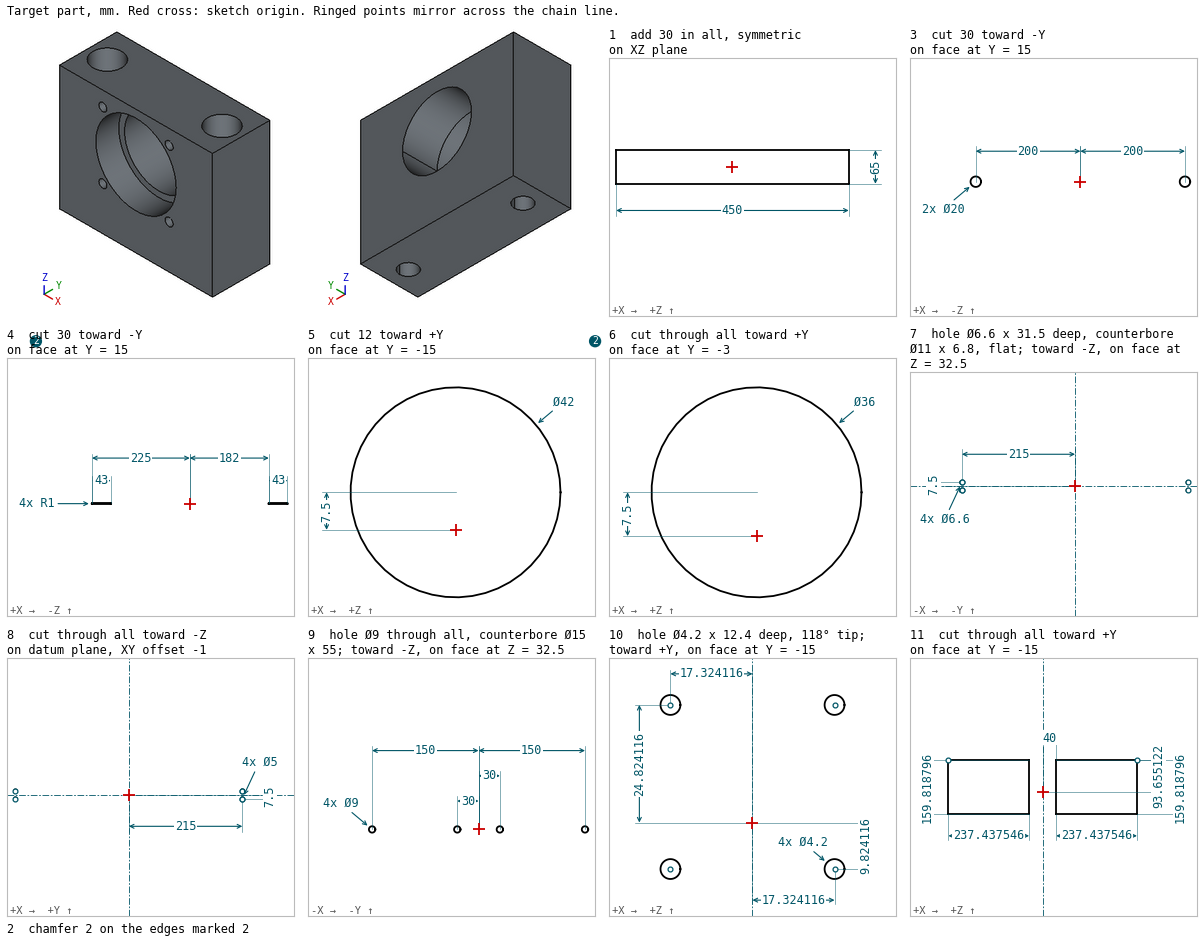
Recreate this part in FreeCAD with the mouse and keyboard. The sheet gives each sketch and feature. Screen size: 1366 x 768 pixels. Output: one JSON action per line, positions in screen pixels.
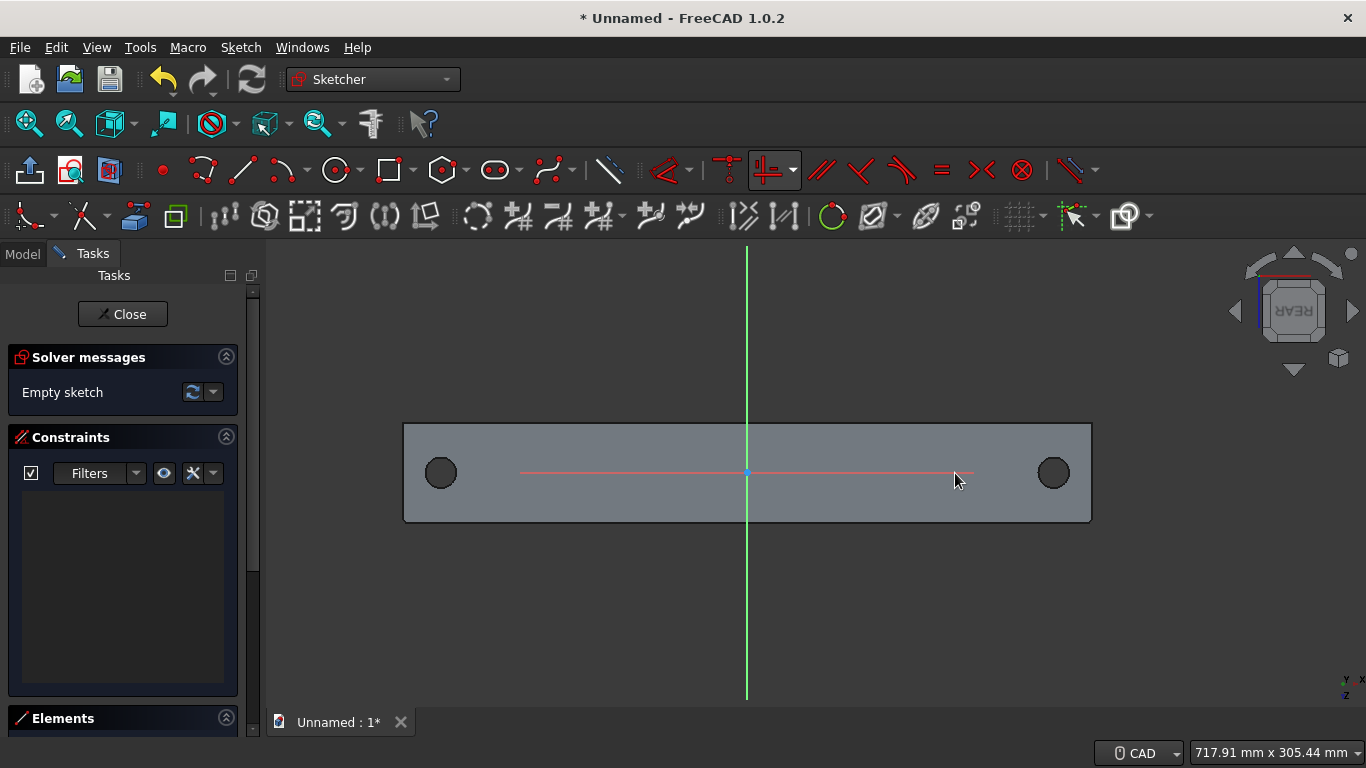
{"action": "scroll", "coordinate": [403, 473], "scroll_direction": "up", "scroll_amount": 14}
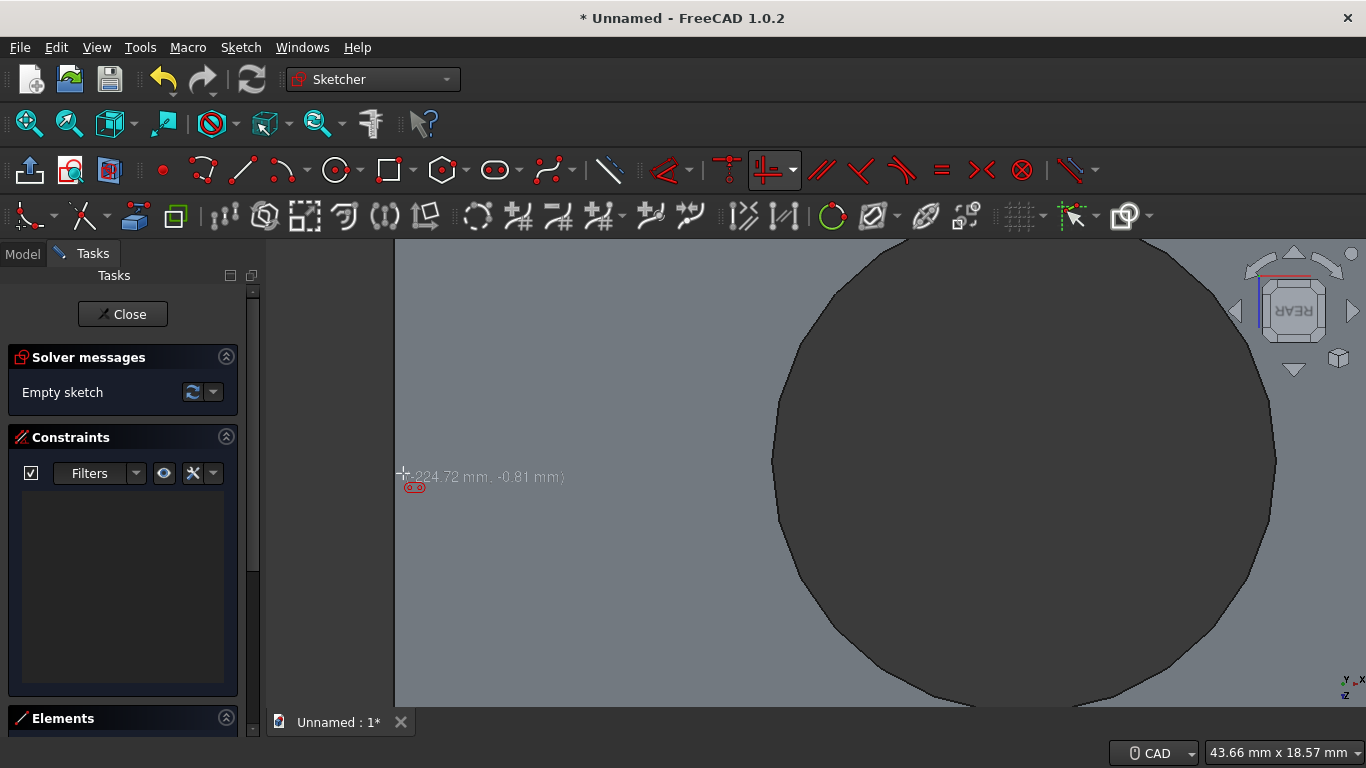
{"action": "scroll", "coordinate": [403, 474], "scroll_direction": "down", "scroll_amount": 14}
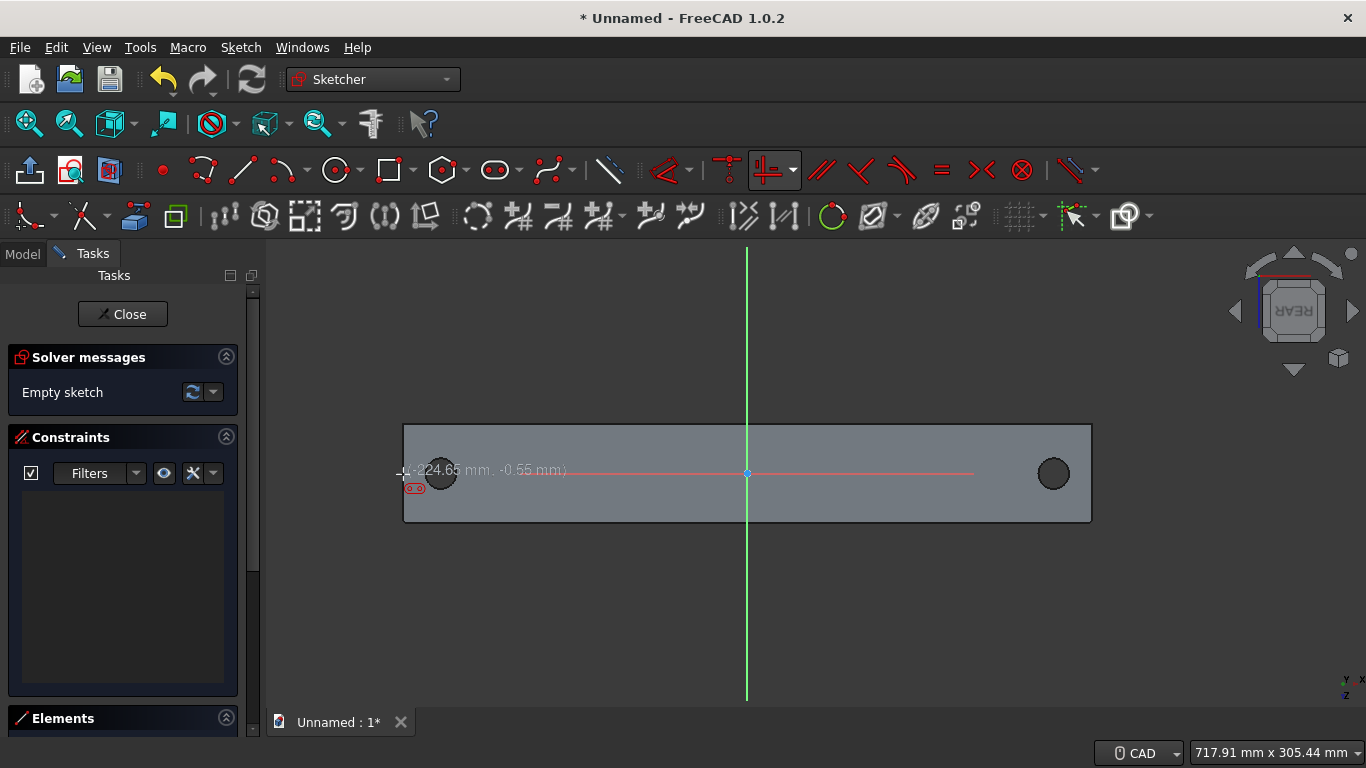
{"action": "left_click", "coordinate": [403, 474]}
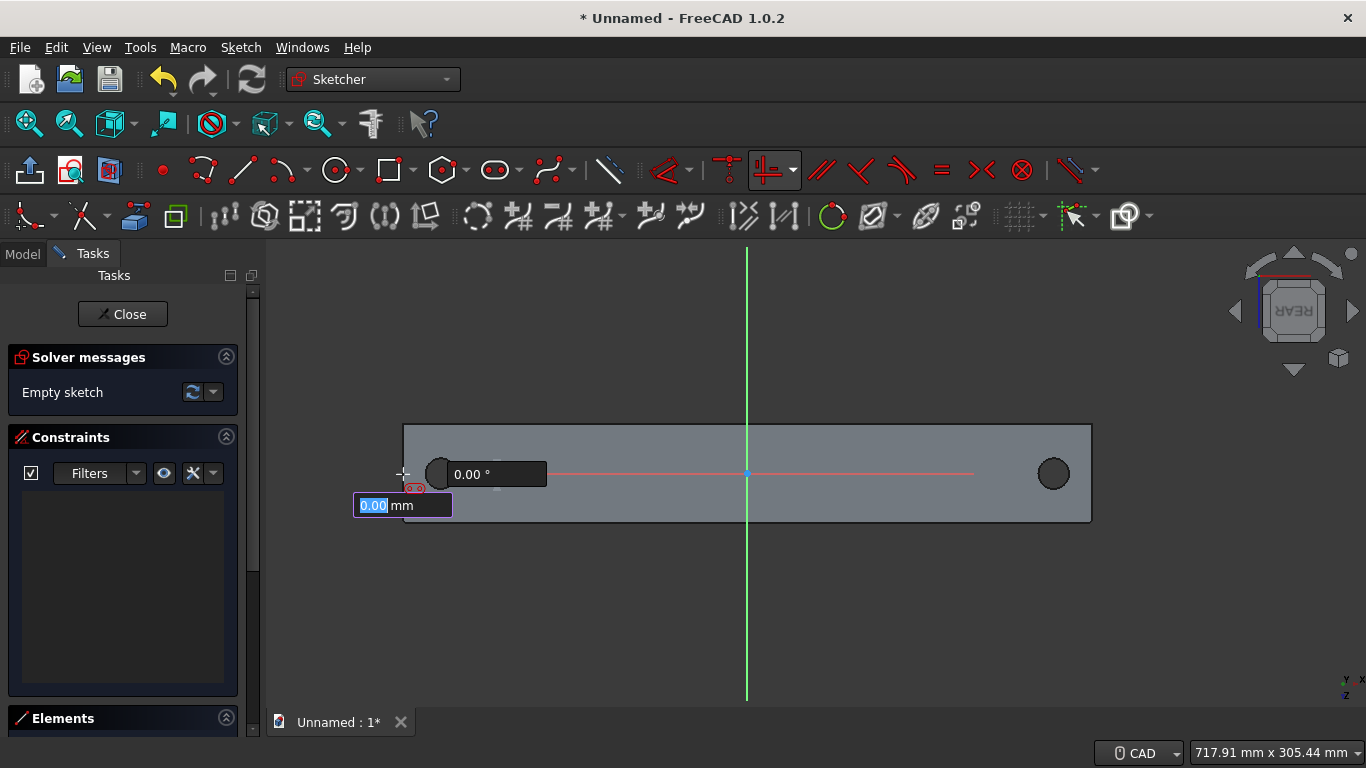
{"action": "left_click", "coordinate": [468, 465]}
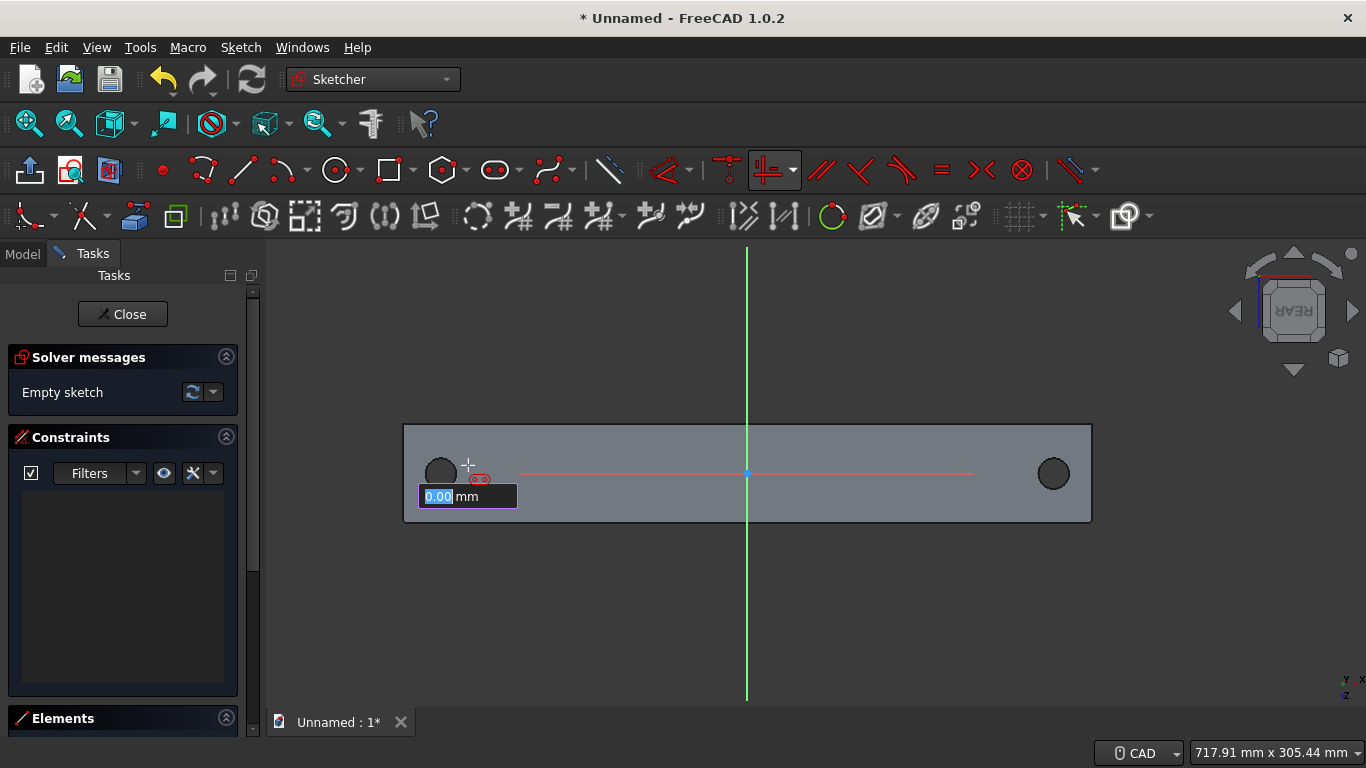
{"action": "scroll", "coordinate": [436, 472], "scroll_direction": "up", "scroll_amount": 12}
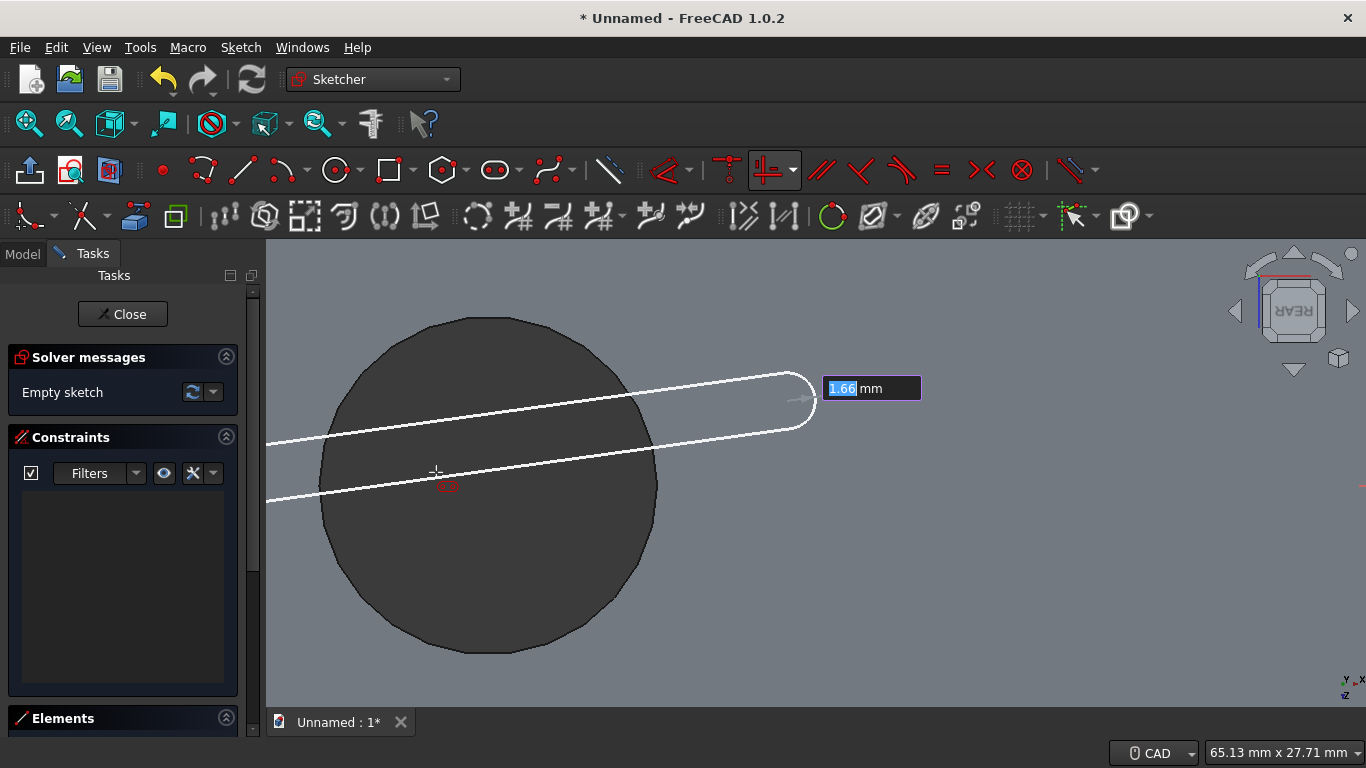
{"action": "left_click", "coordinate": [429, 469]}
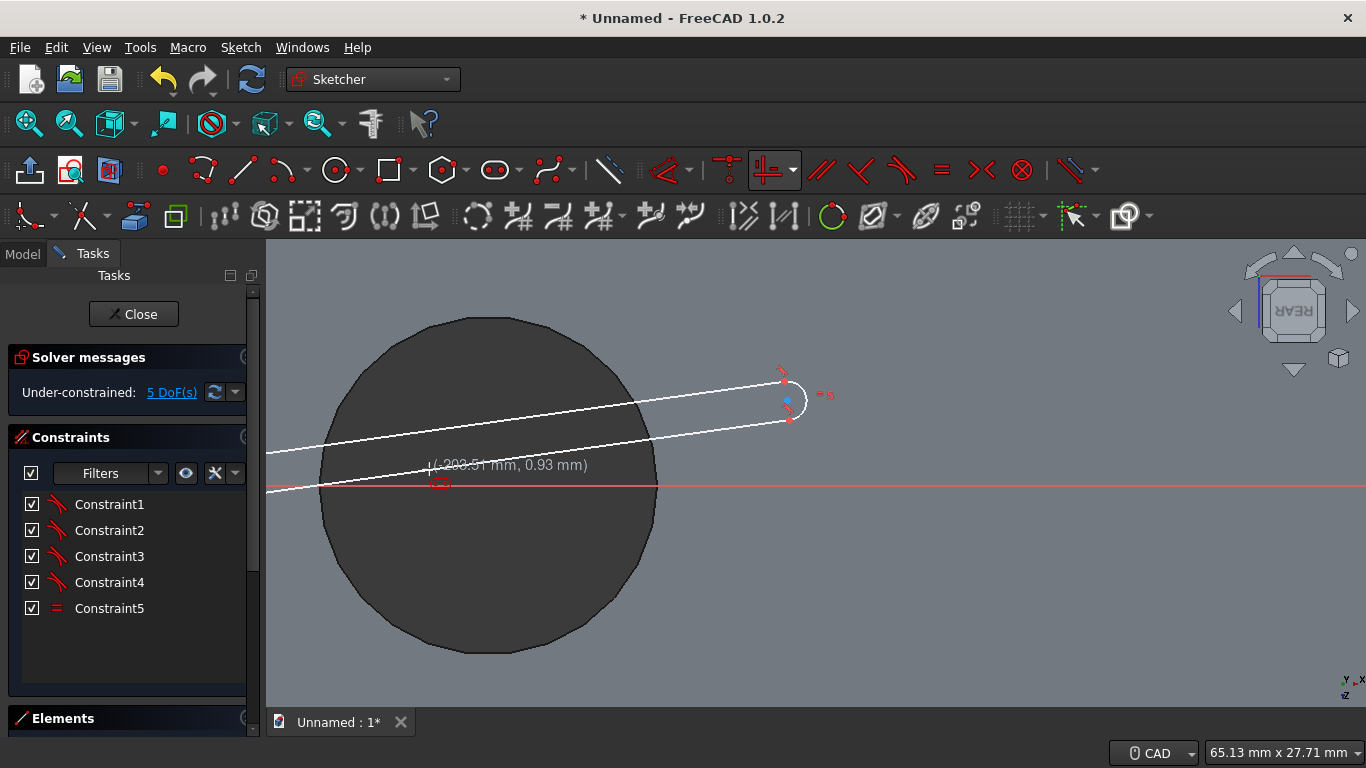
{"action": "scroll", "coordinate": [436, 472], "scroll_direction": "down", "scroll_amount": 12}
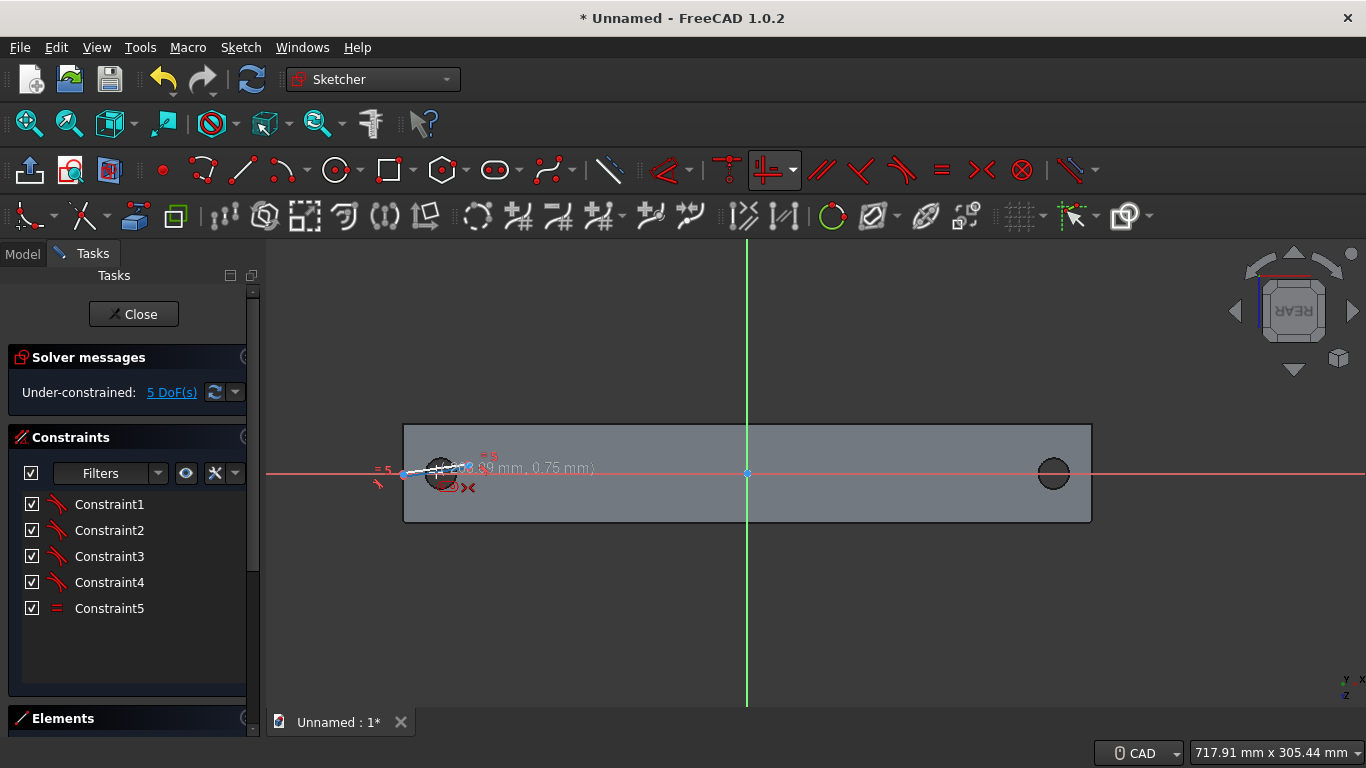
{"action": "scroll", "coordinate": [1026, 474], "scroll_direction": "up", "scroll_amount": 14}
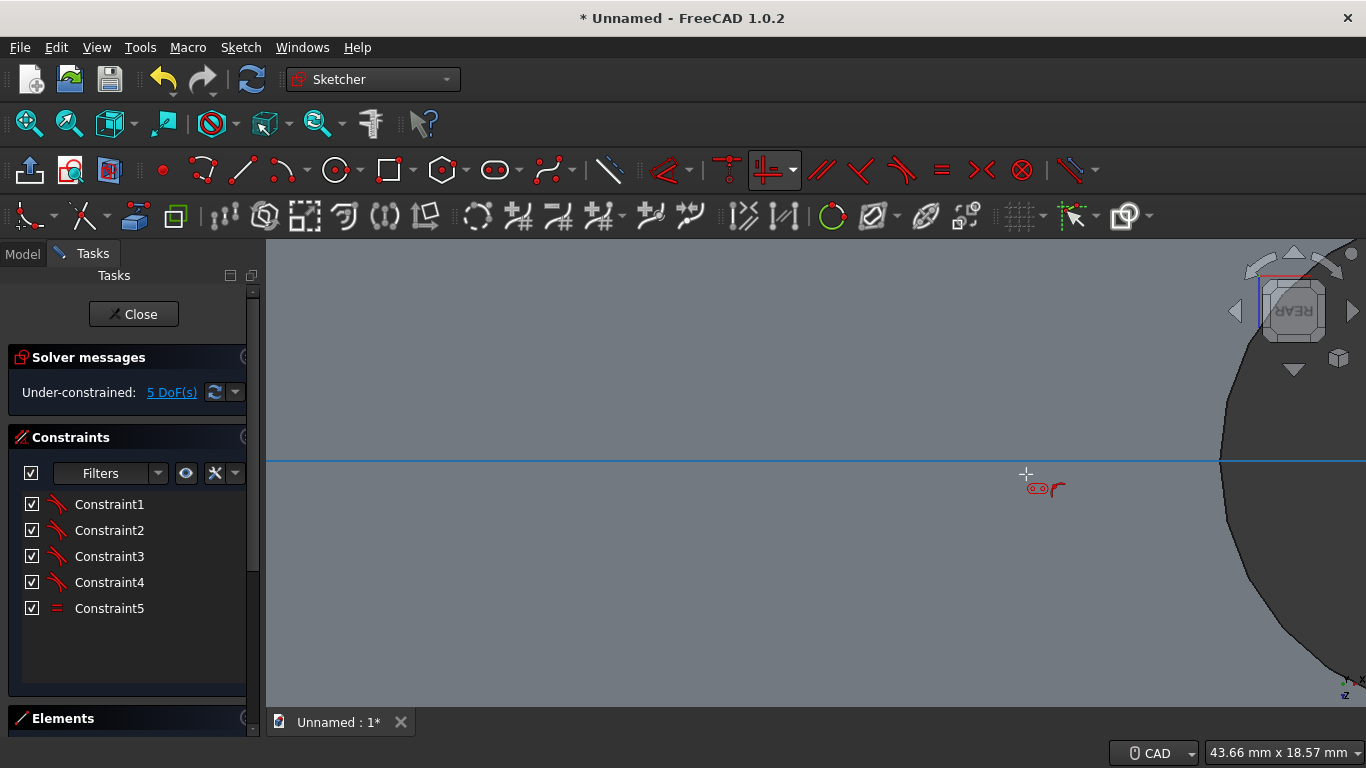
{"action": "scroll", "coordinate": [1027, 474], "scroll_direction": "down", "scroll_amount": 14}